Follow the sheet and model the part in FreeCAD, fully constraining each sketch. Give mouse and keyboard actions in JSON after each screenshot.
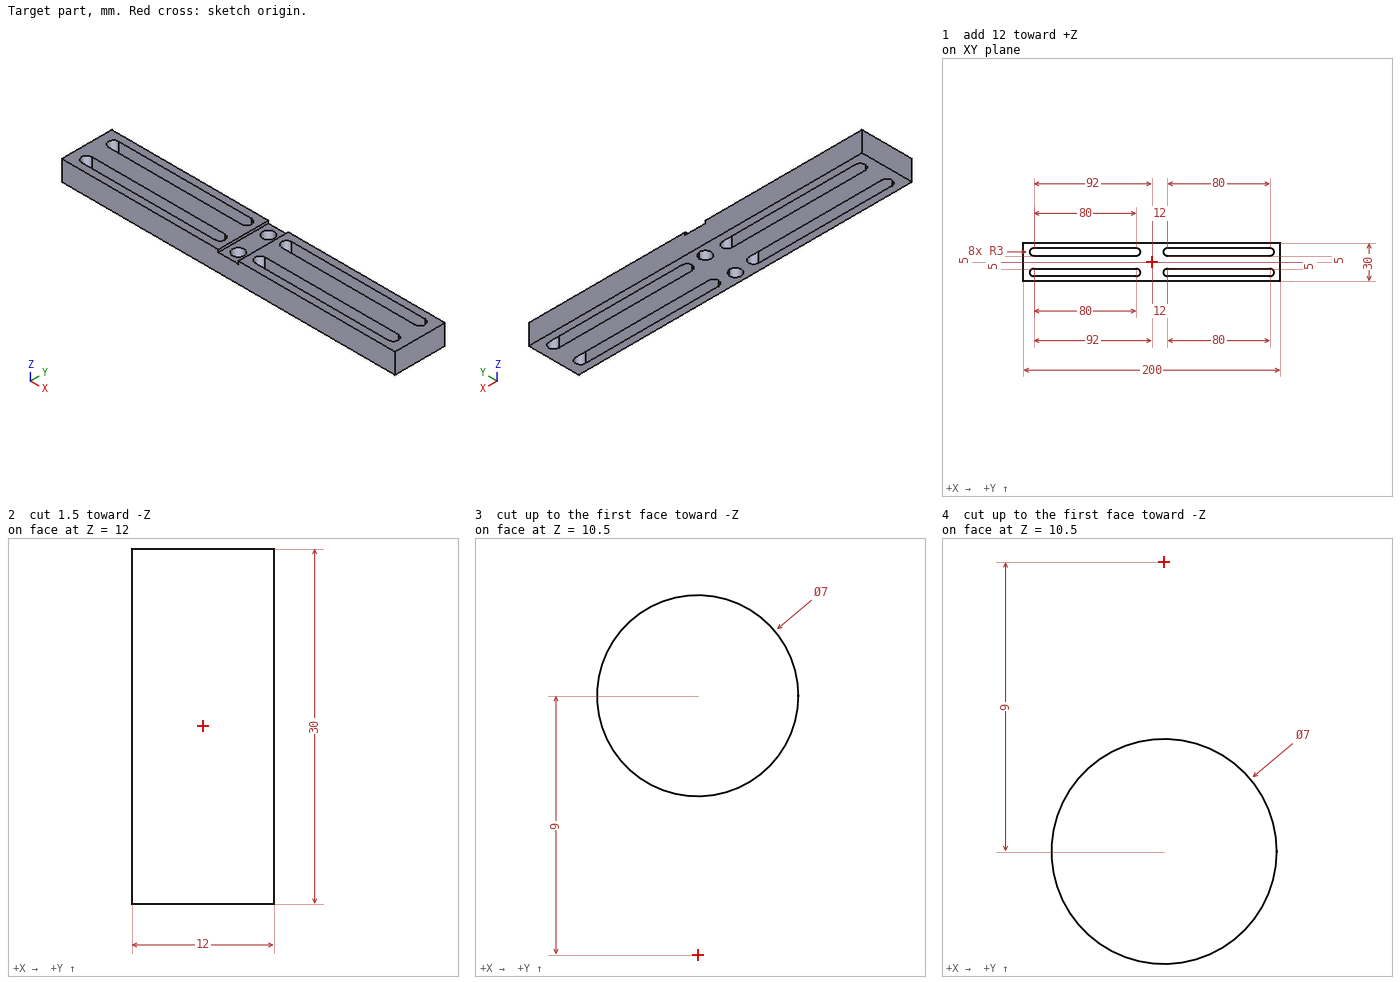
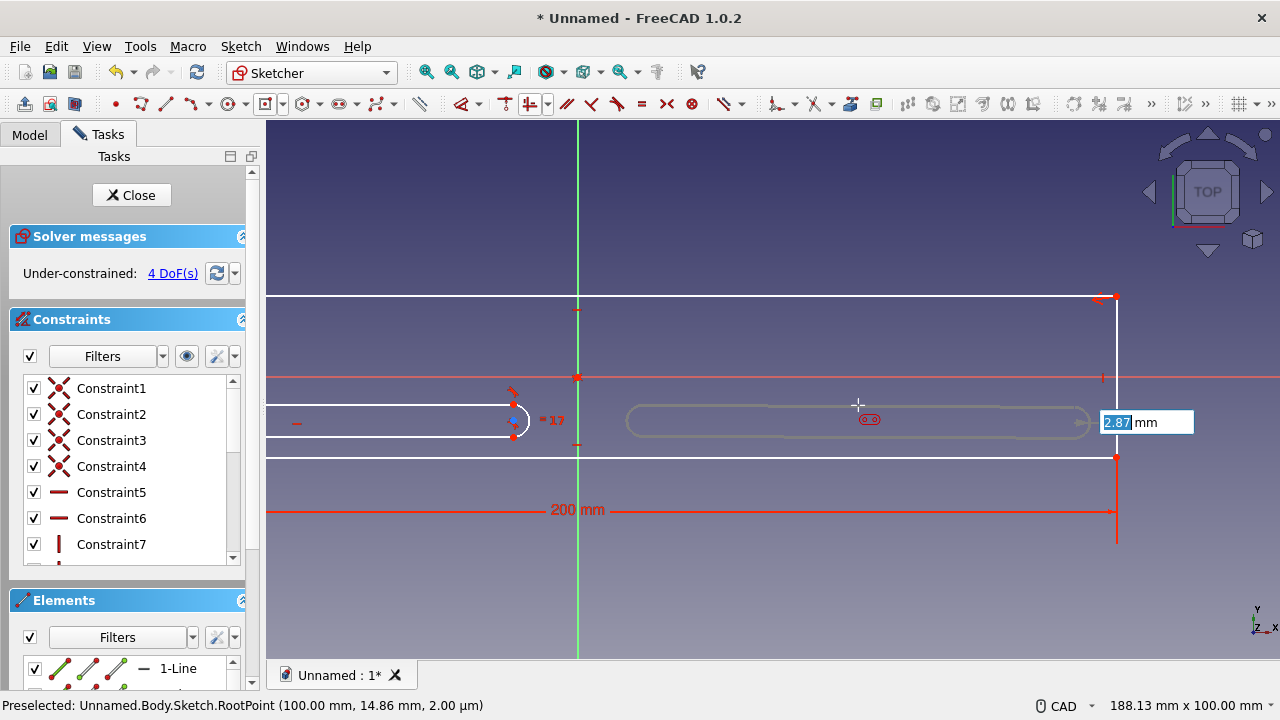
{"action": "left_click", "coordinate": [858, 404]}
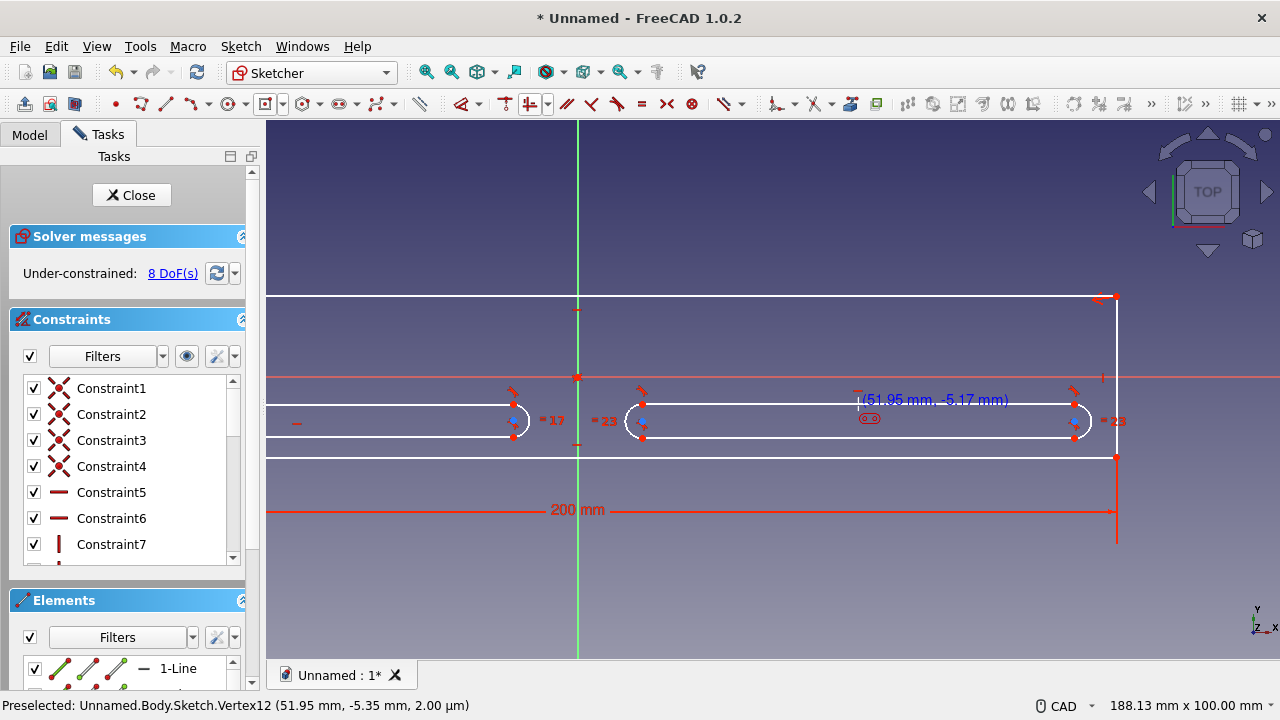
{"action": "scroll", "coordinate": [858, 405], "scroll_direction": "down", "scroll_amount": 3}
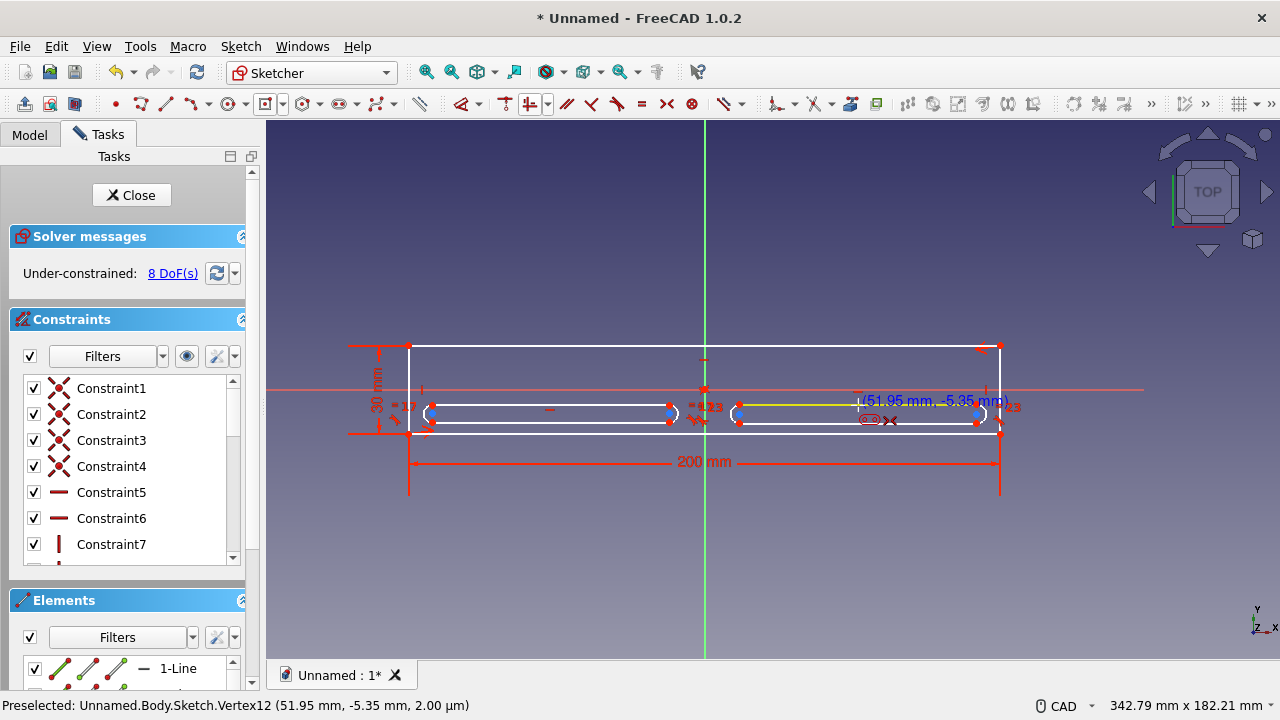
{"action": "scroll", "coordinate": [432, 366], "scroll_direction": "up", "scroll_amount": 5}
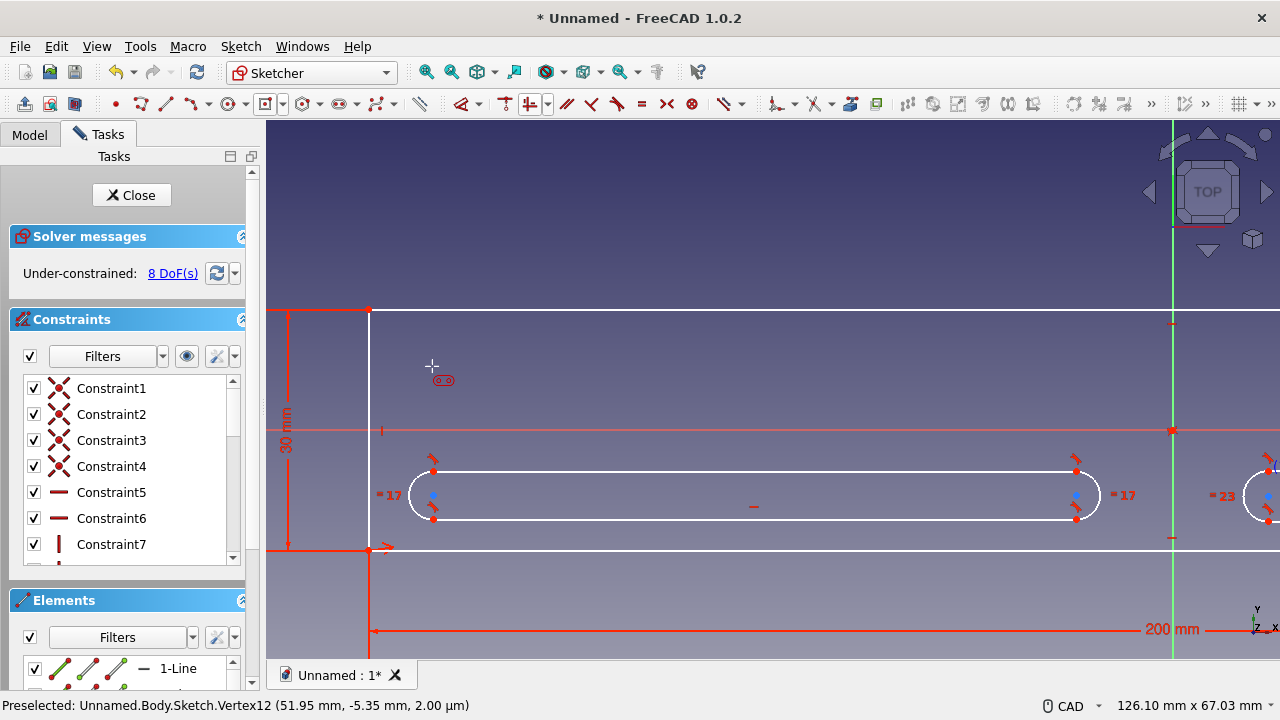
{"action": "left_click", "coordinate": [433, 366]}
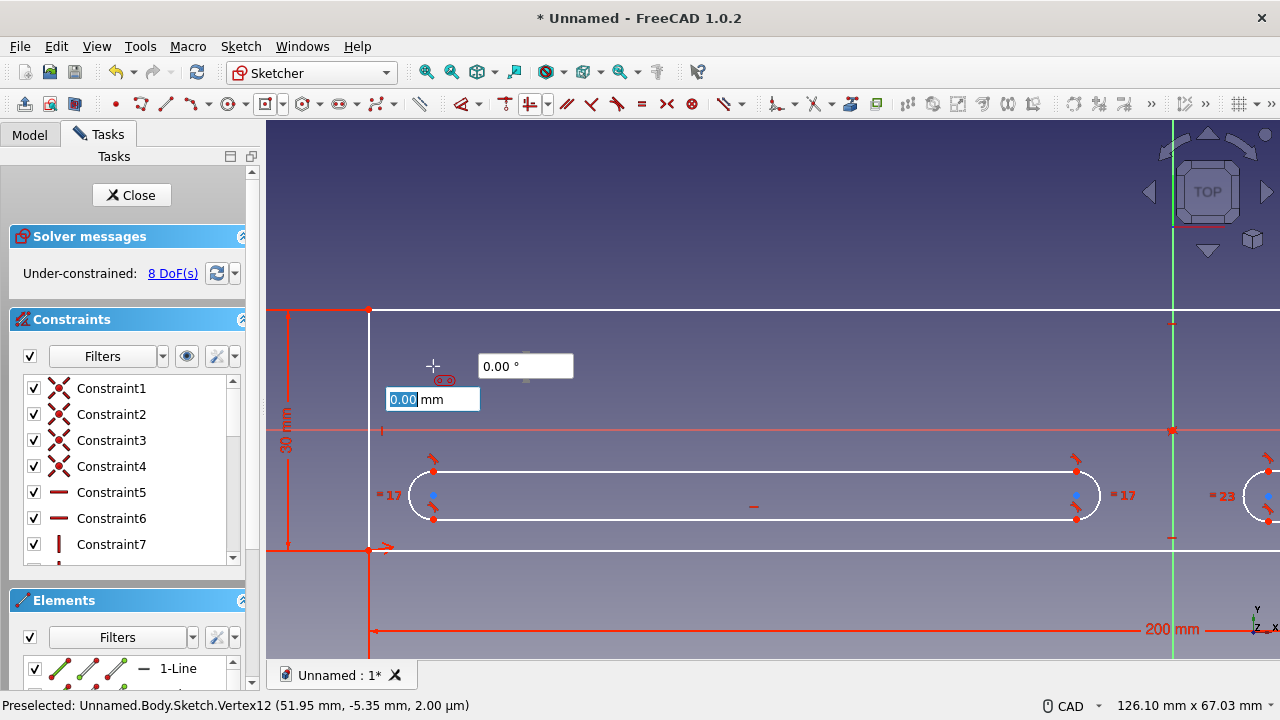
{"action": "left_click", "coordinate": [1076, 366]}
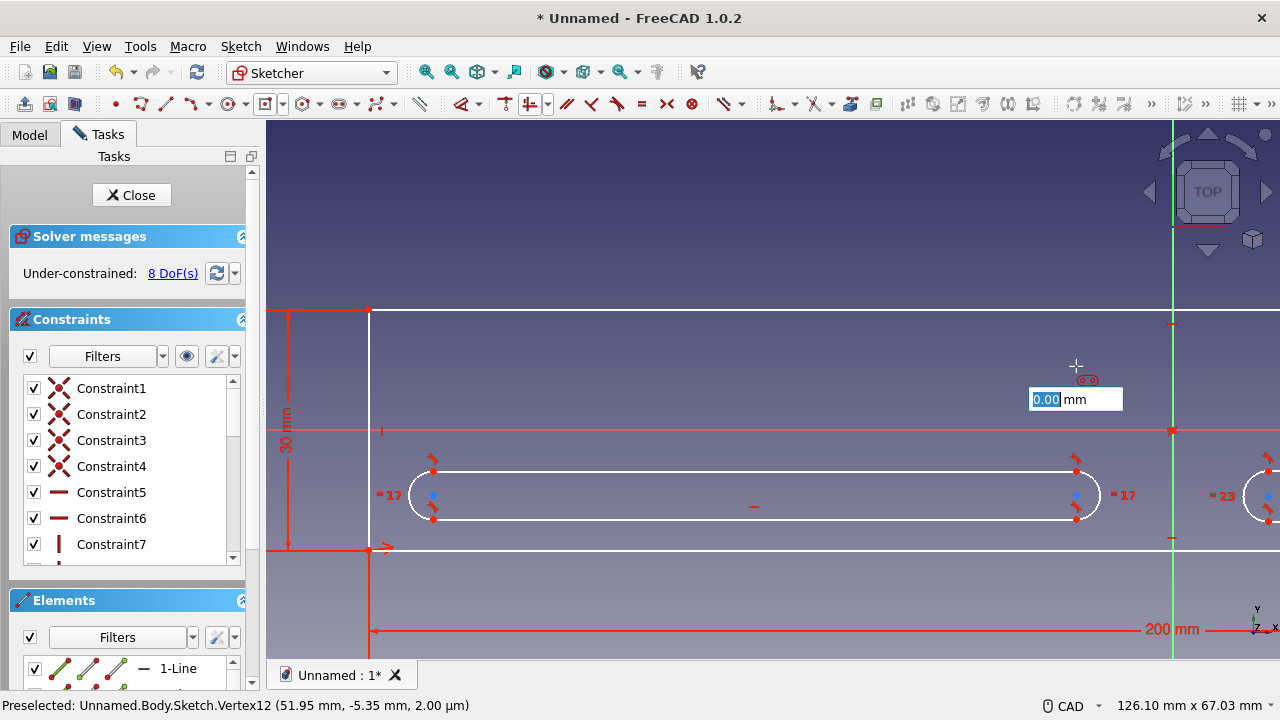
{"action": "left_click", "coordinate": [755, 342]}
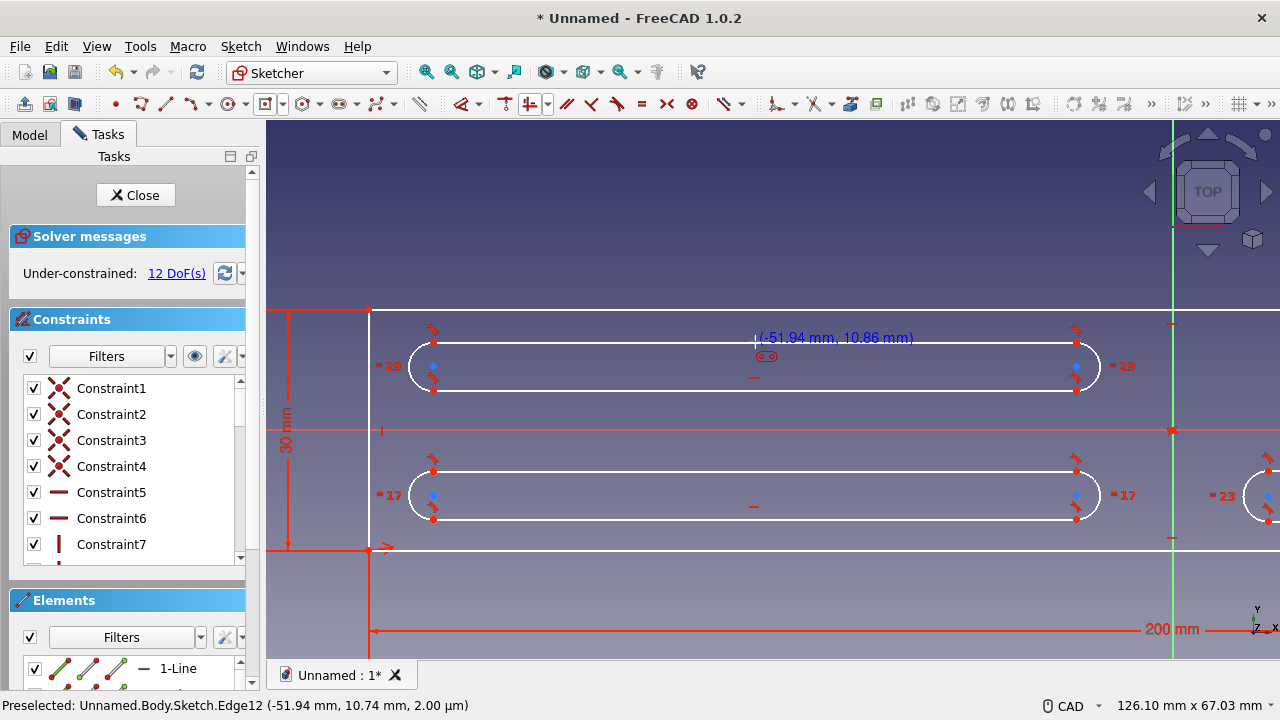
{"action": "scroll", "coordinate": [432, 366], "scroll_direction": "down", "scroll_amount": 5}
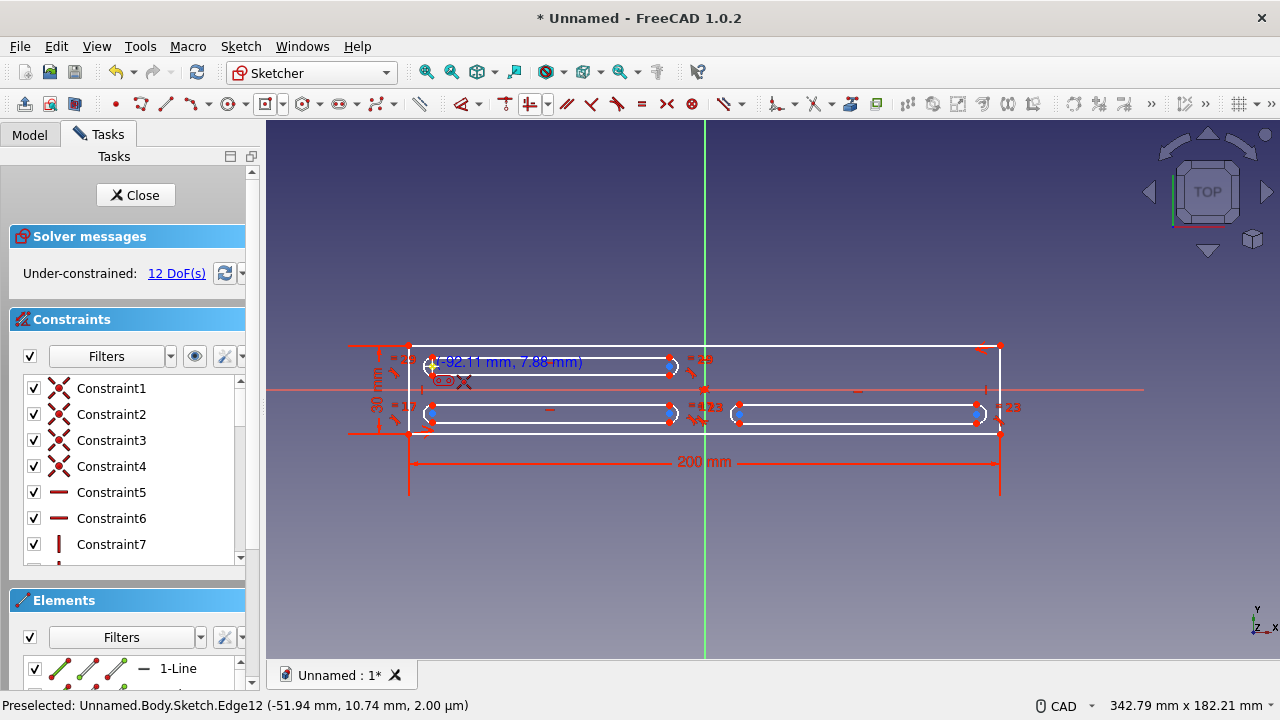
{"action": "scroll", "coordinate": [740, 366], "scroll_direction": "up", "scroll_amount": 5}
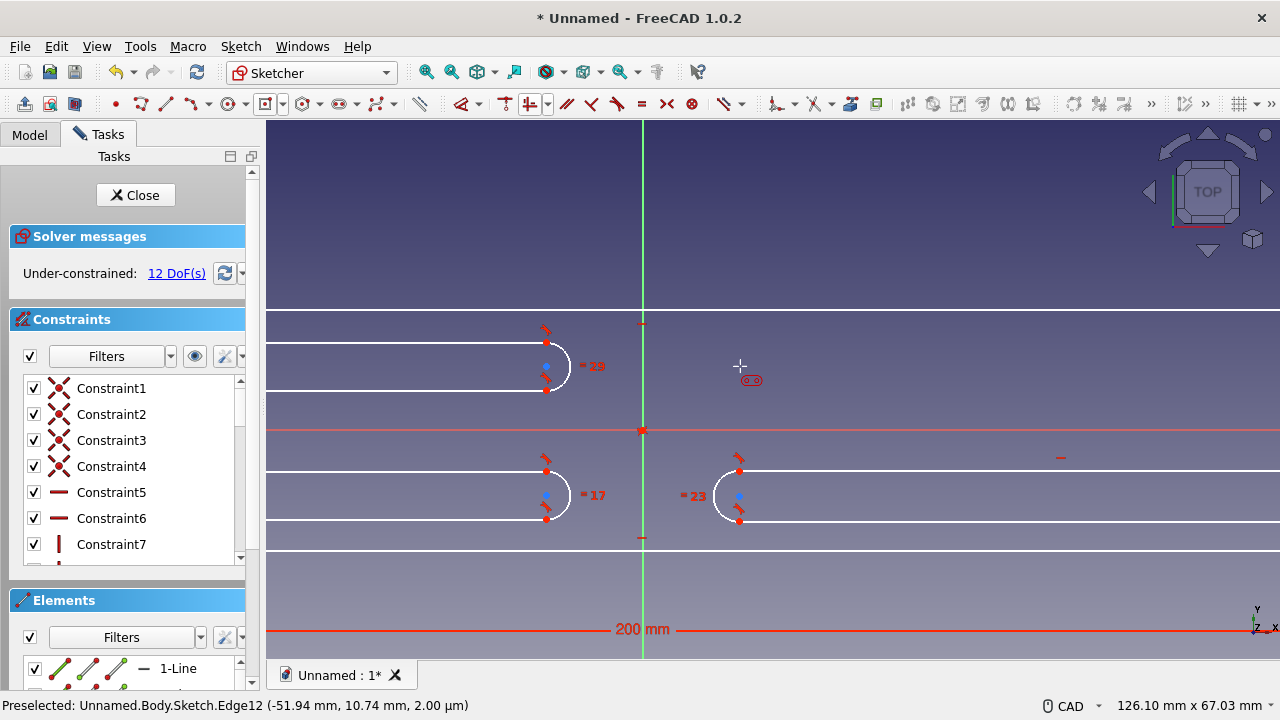
{"action": "left_click", "coordinate": [739, 366]}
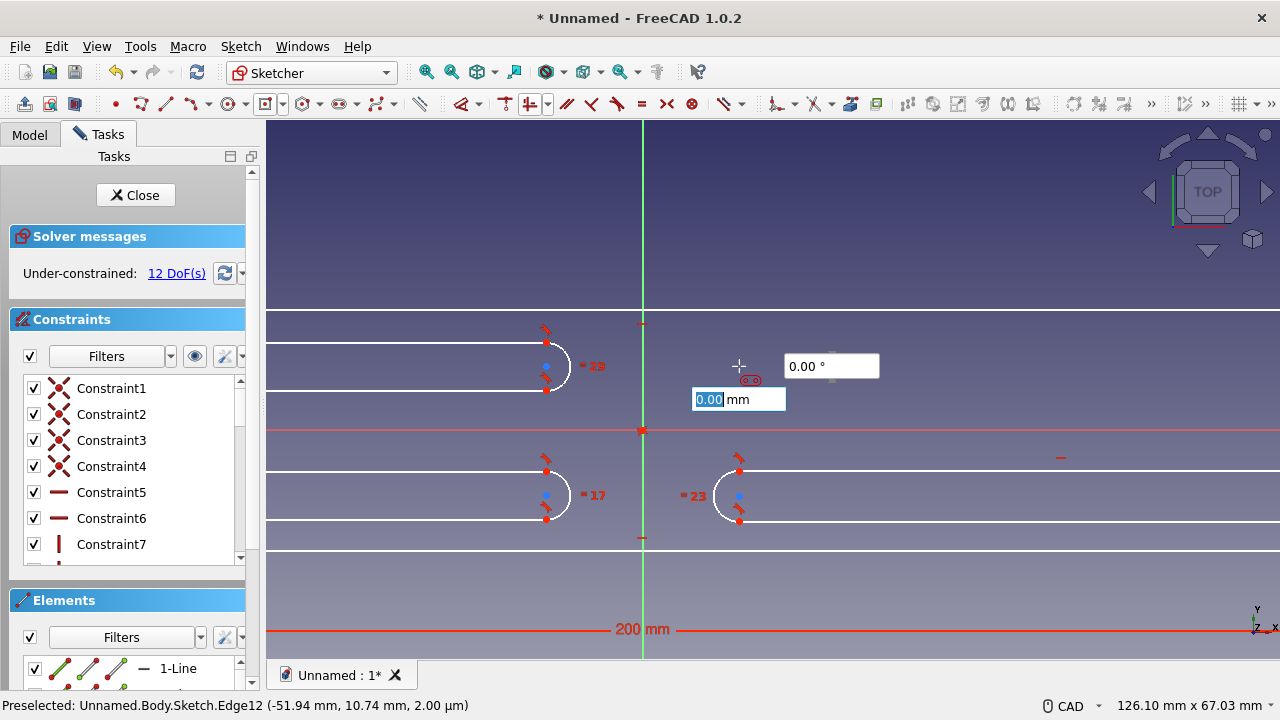
{"action": "scroll", "coordinate": [740, 366], "scroll_direction": "down", "scroll_amount": 5}